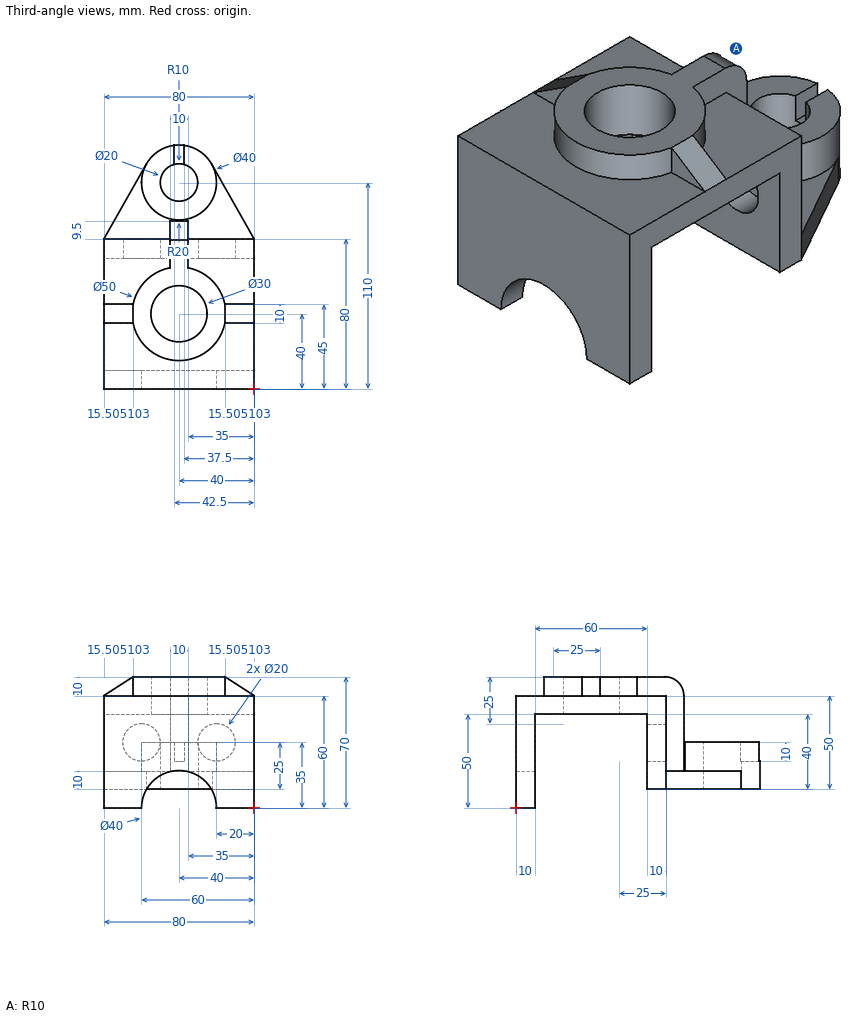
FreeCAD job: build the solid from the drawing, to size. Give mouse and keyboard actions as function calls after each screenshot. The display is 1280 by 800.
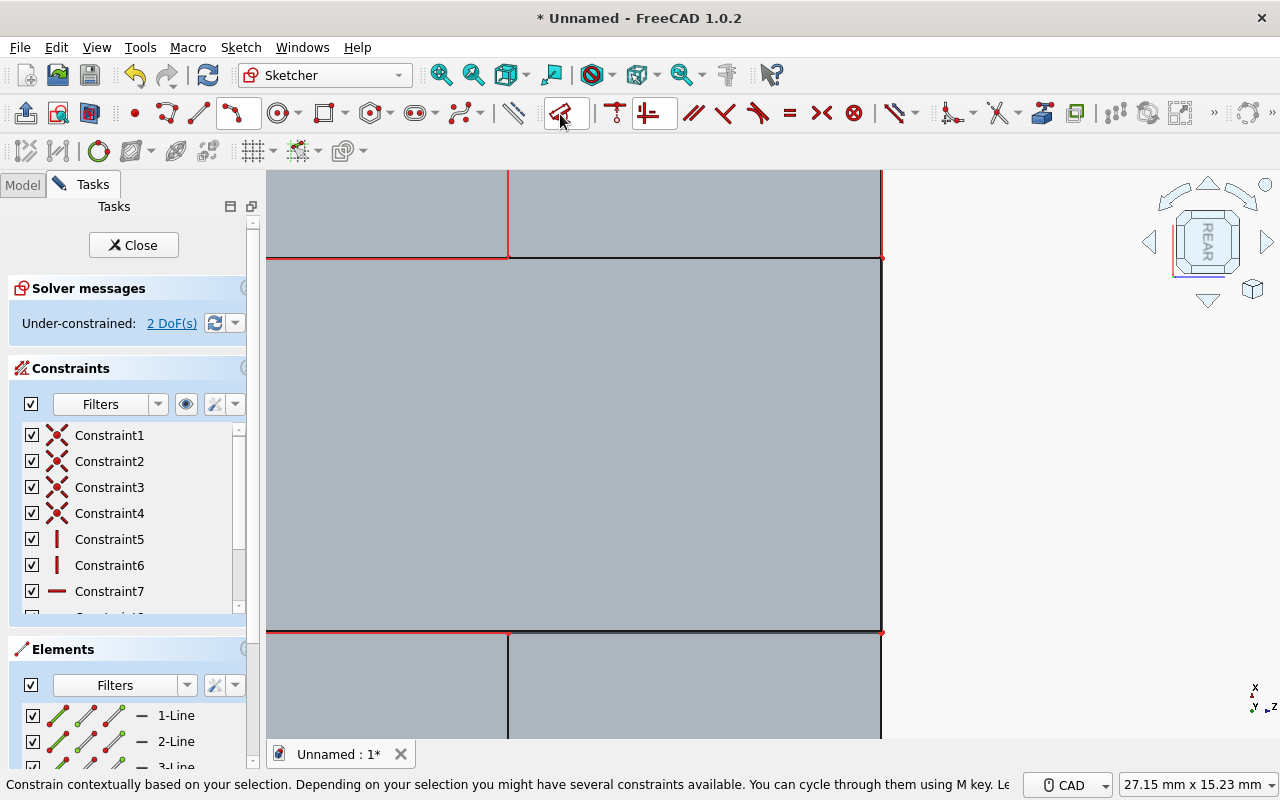
click(508, 259)
click(401, 293)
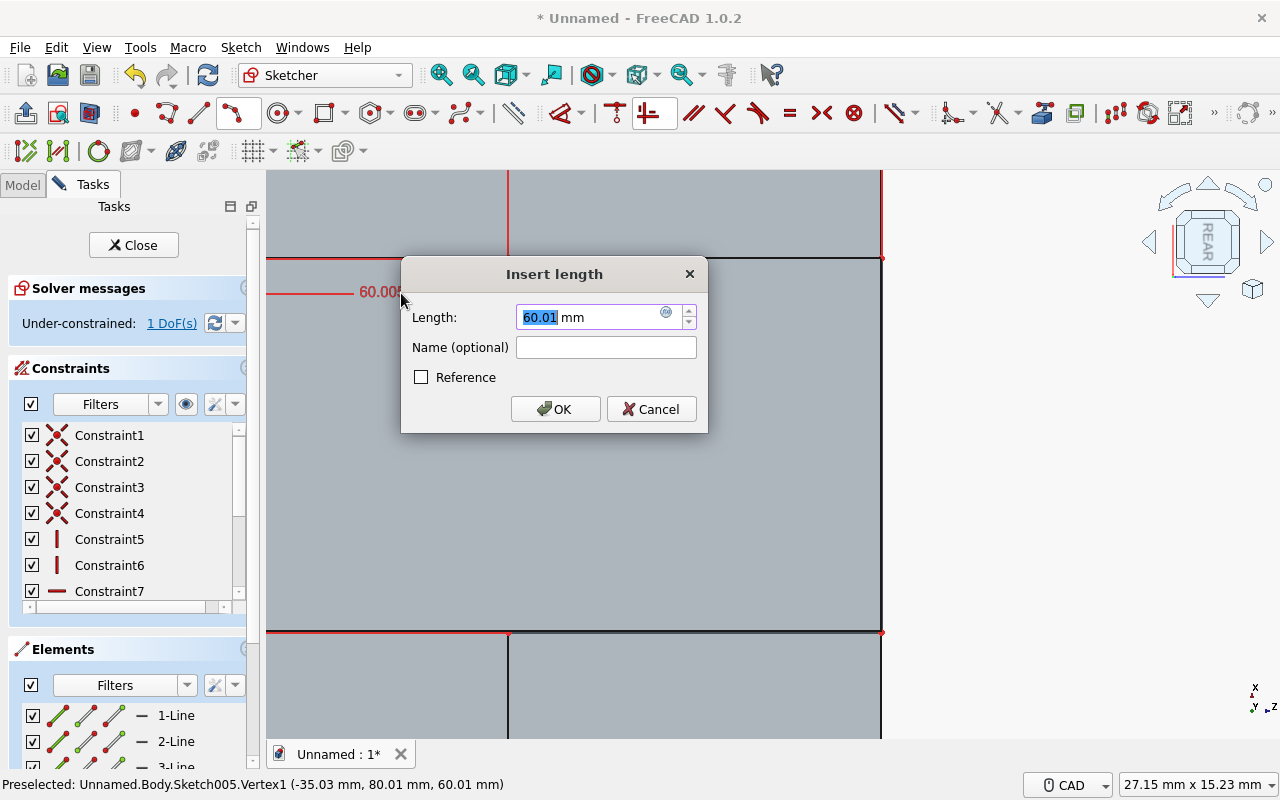
text(60)
key(Return)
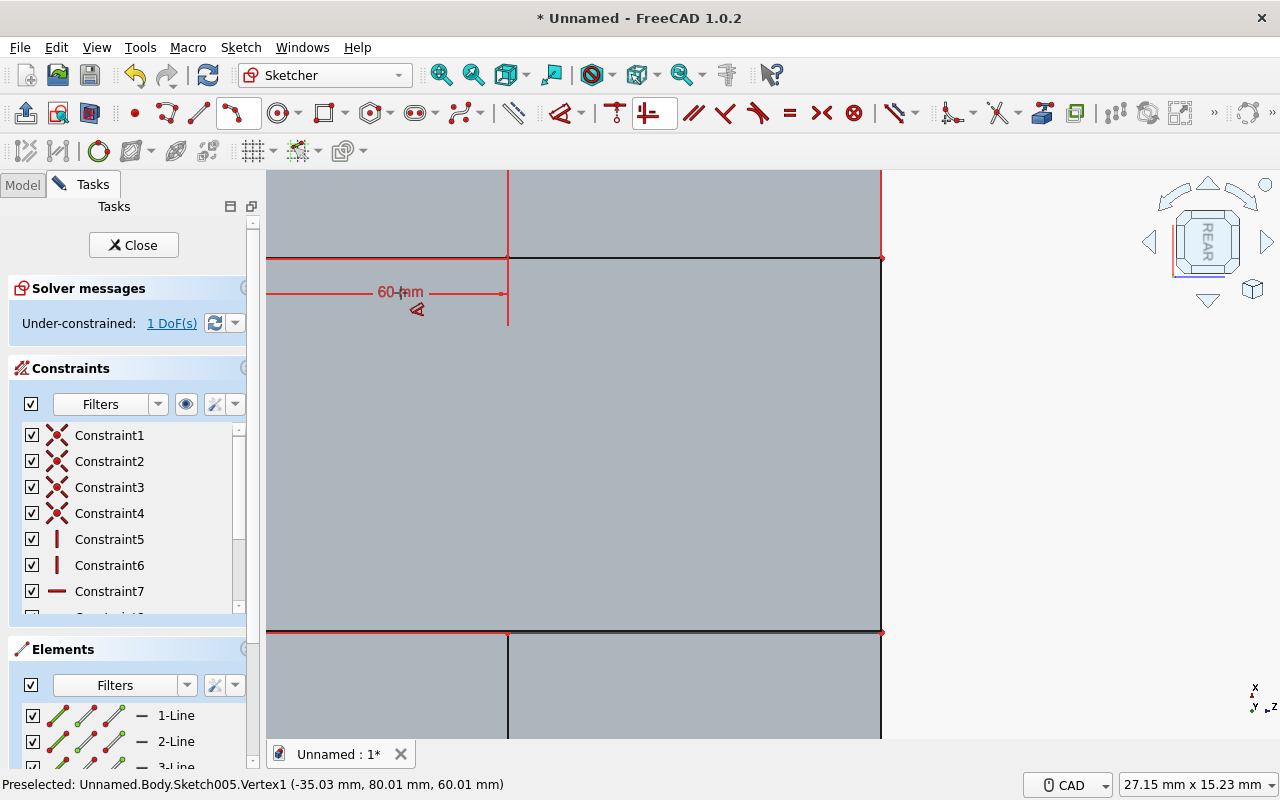
click(508, 259)
click(542, 228)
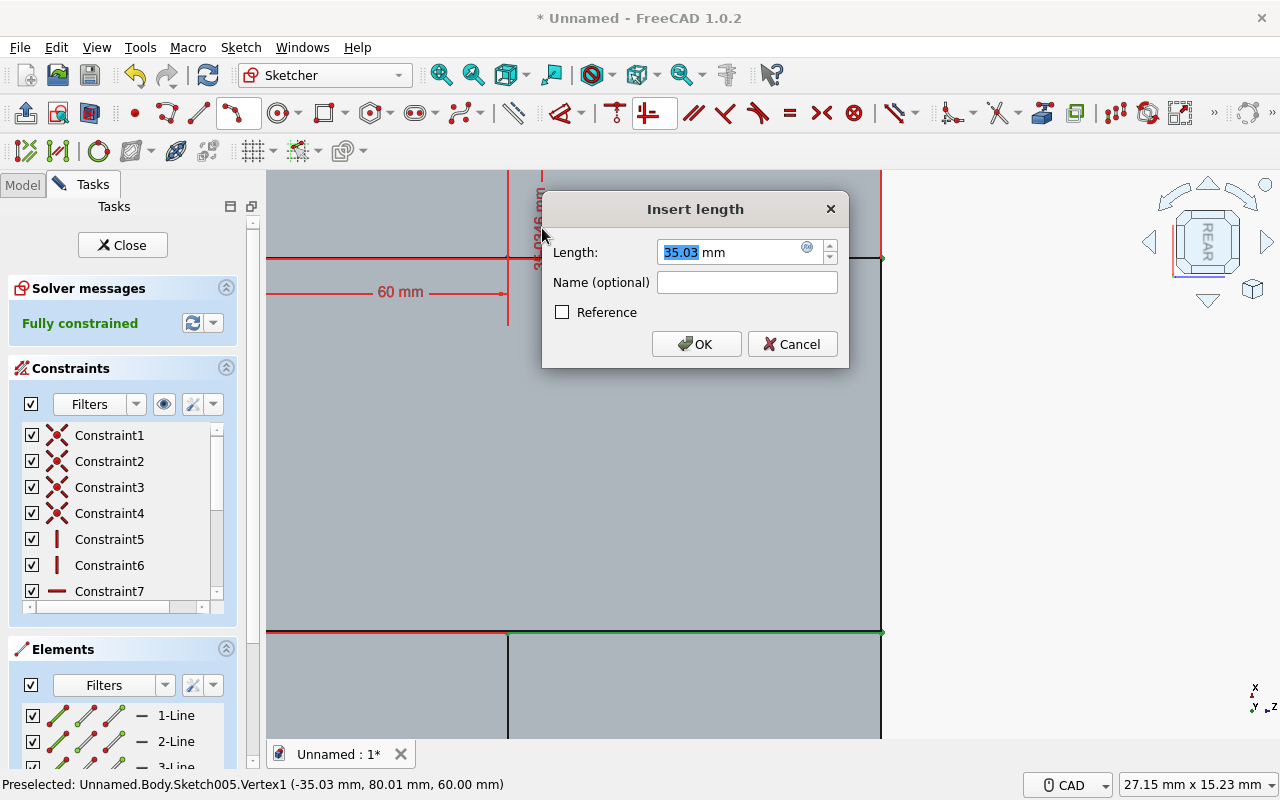
text(35)
key(Return)
key(Escape)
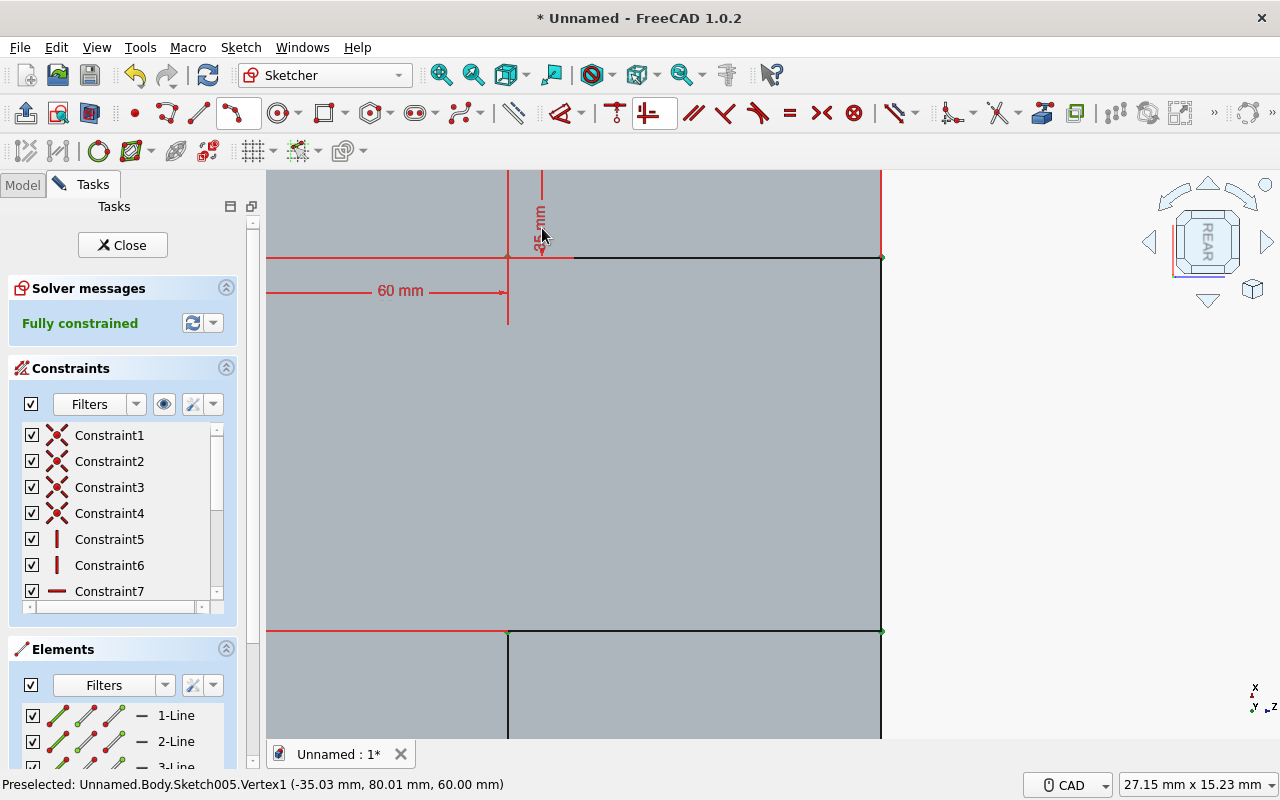
click(123, 245)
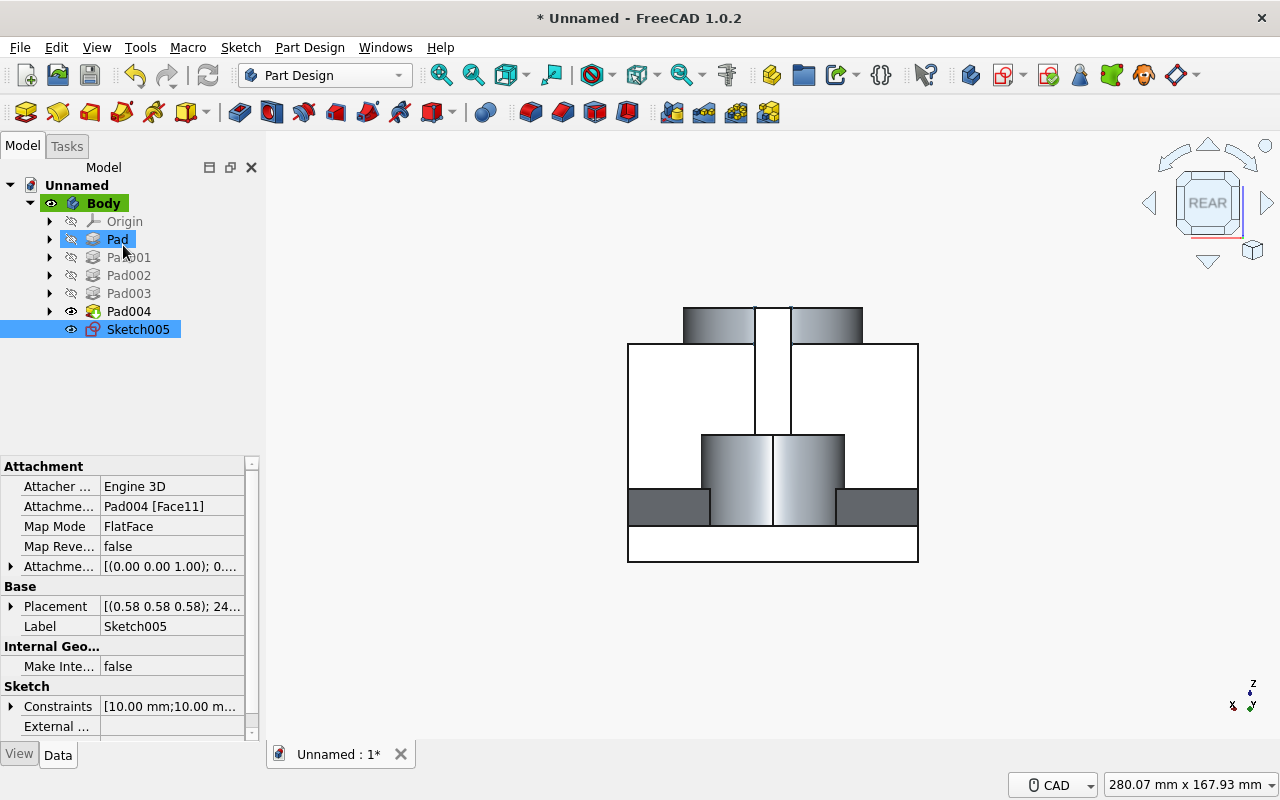
click(26, 112)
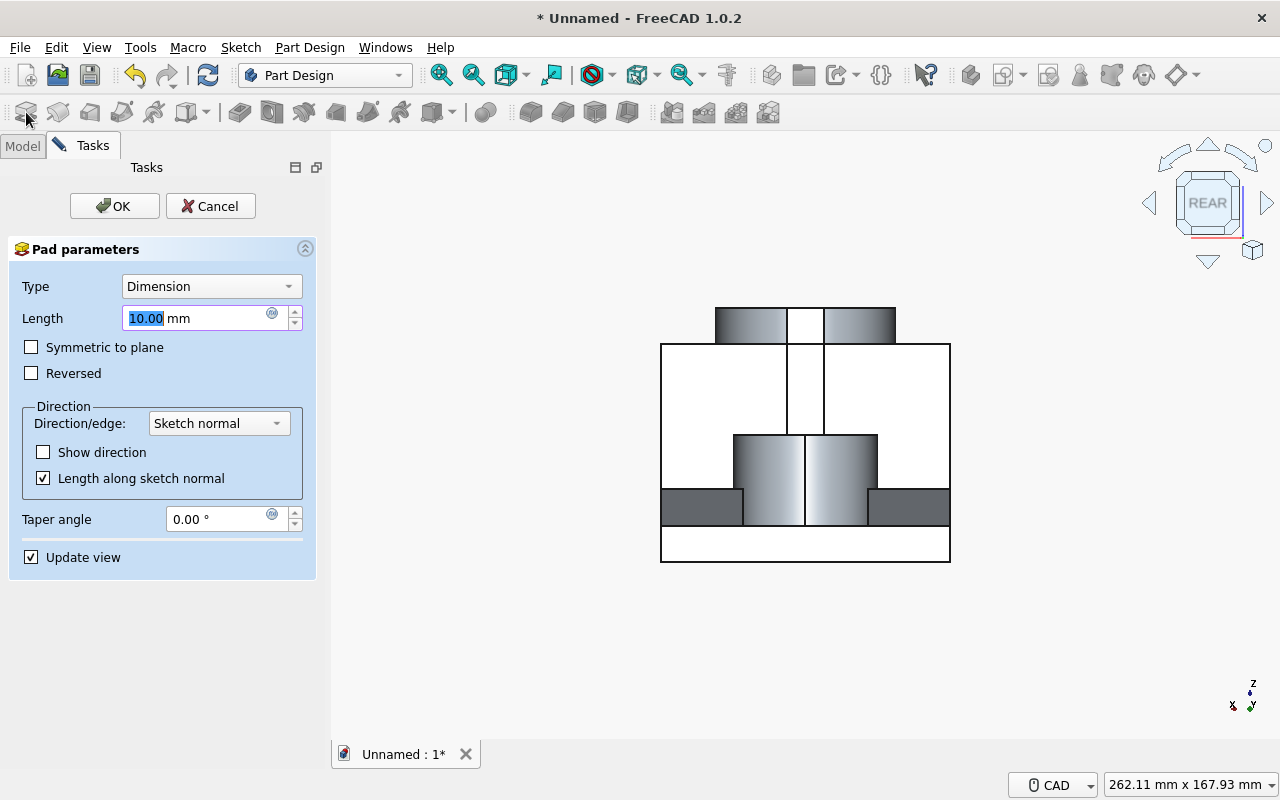
click(212, 286)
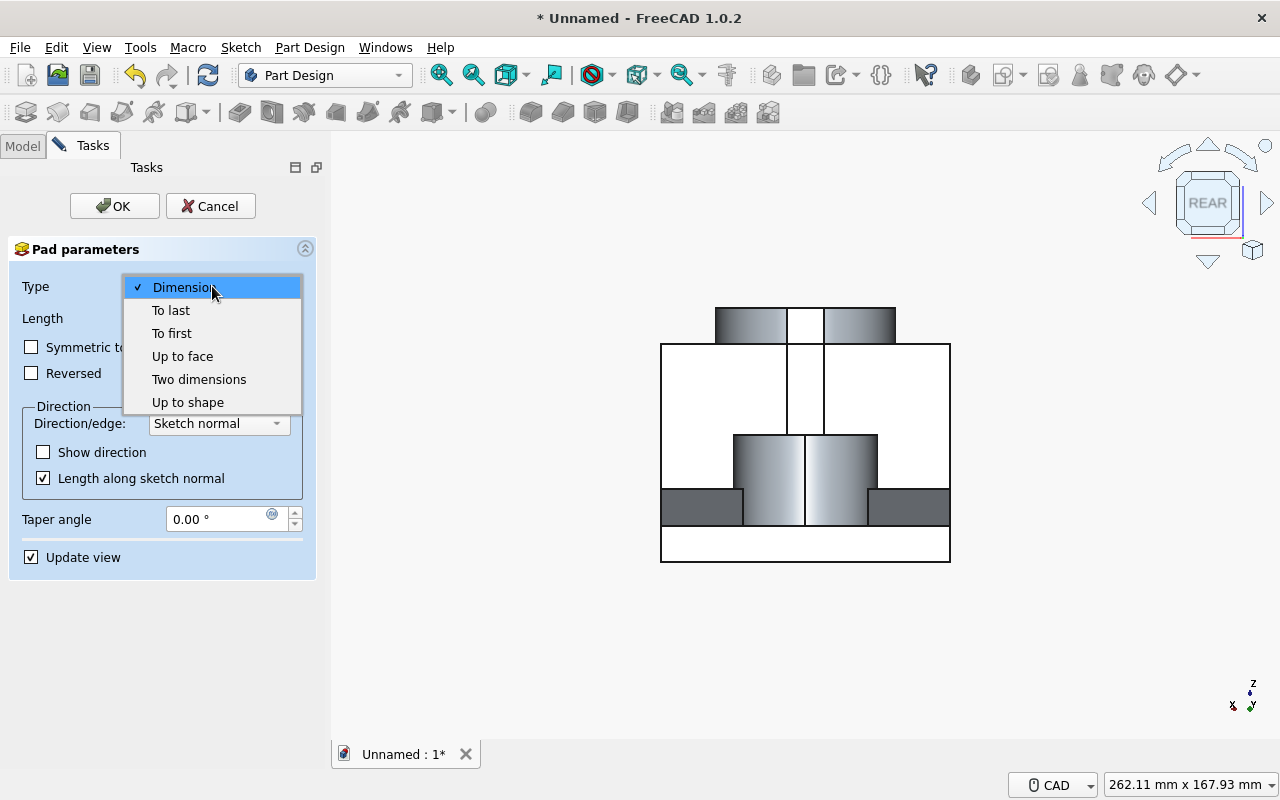
click(212, 334)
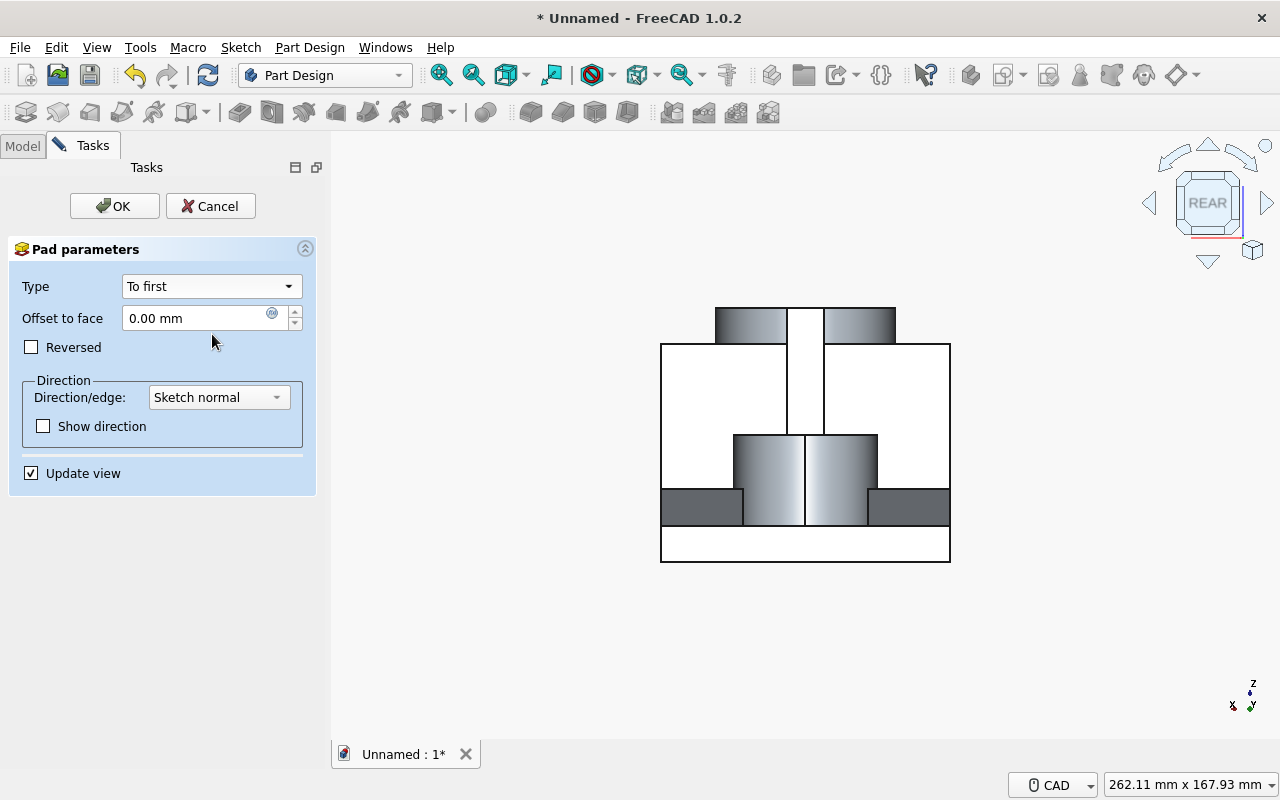
click(30, 347)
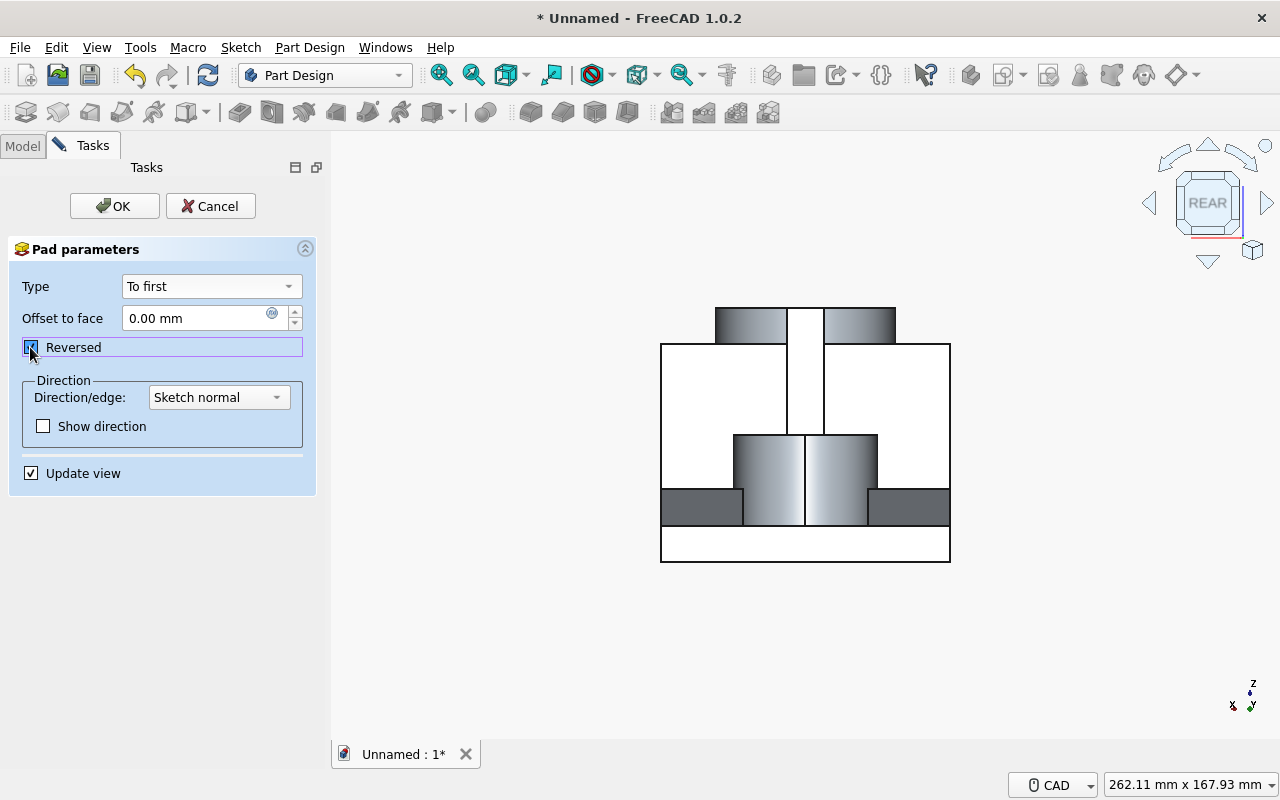
click(115, 206)